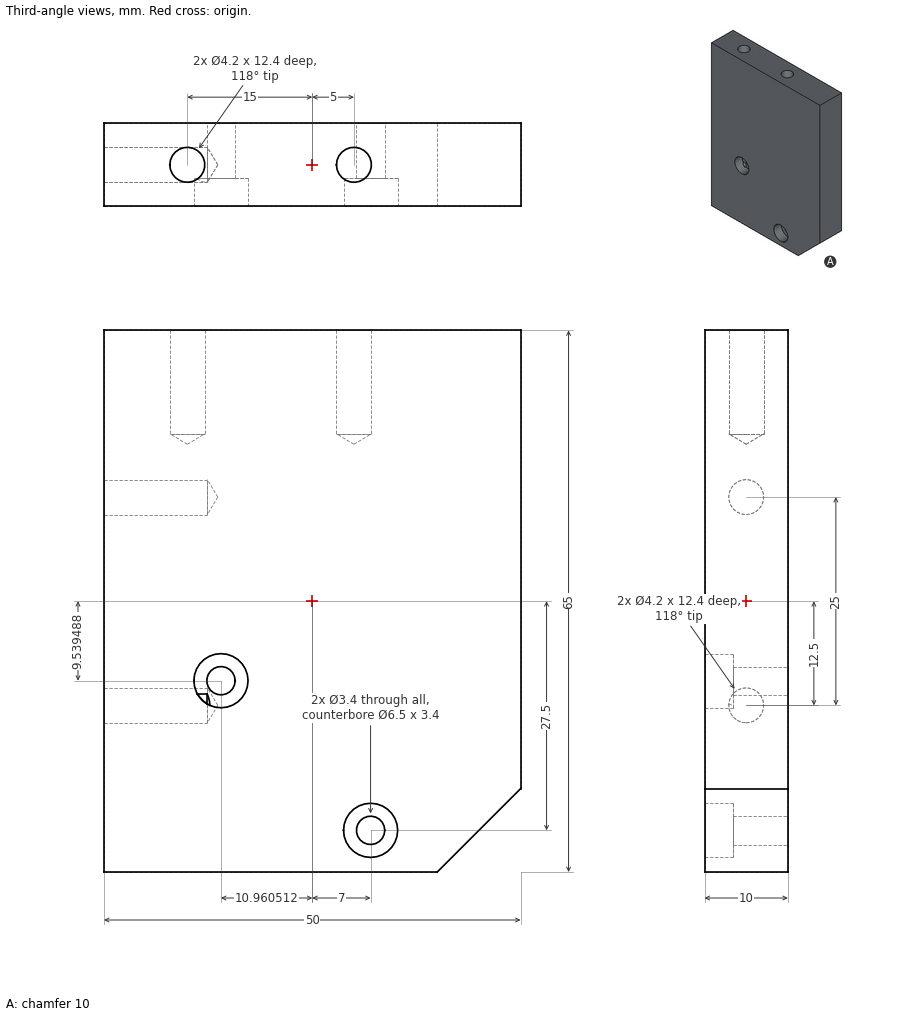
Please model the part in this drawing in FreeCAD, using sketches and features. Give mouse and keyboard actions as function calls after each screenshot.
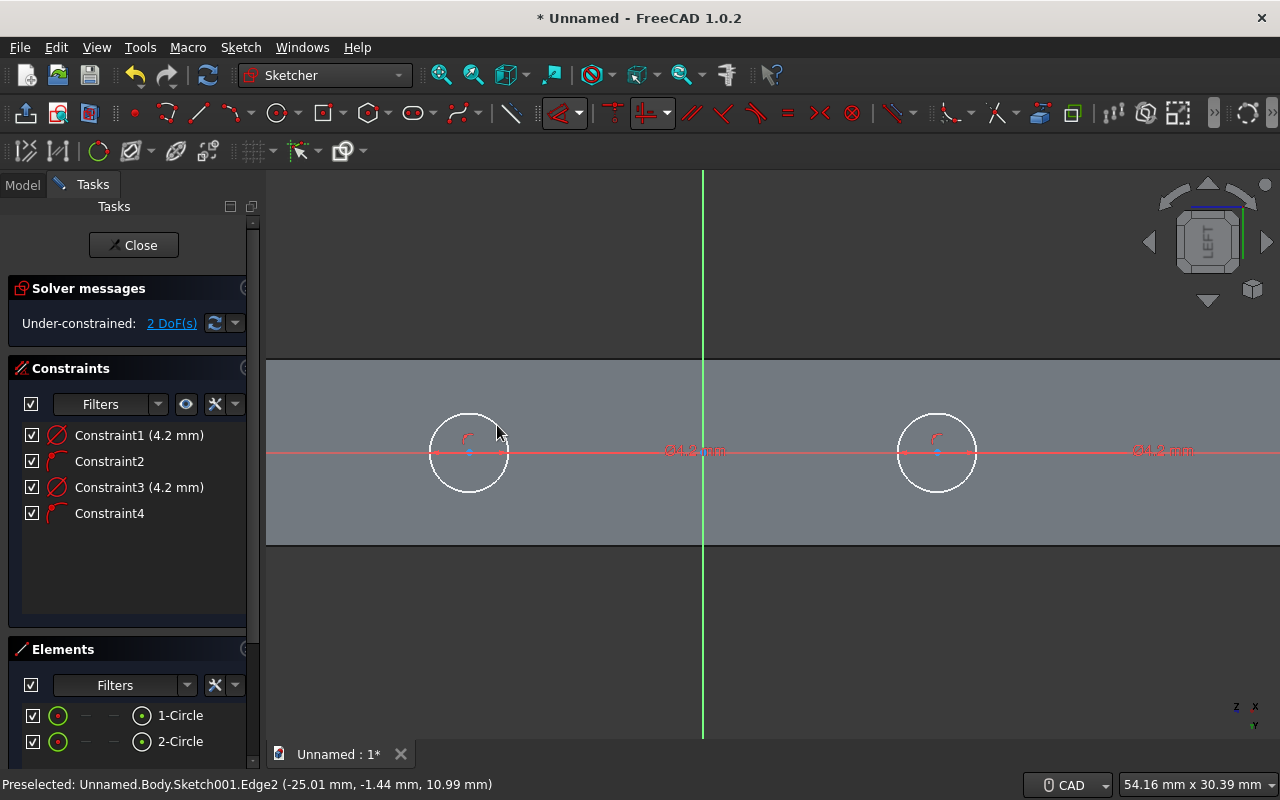
key(d)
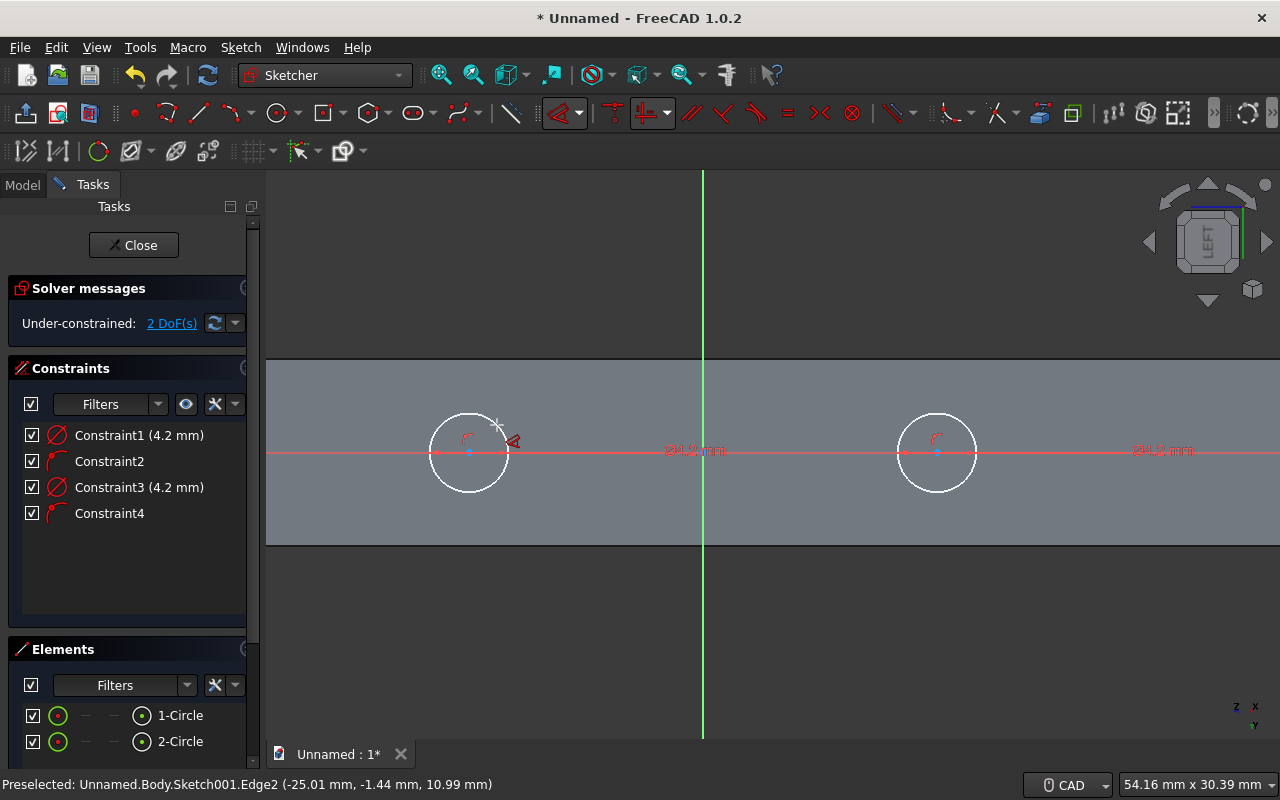
click(937, 453)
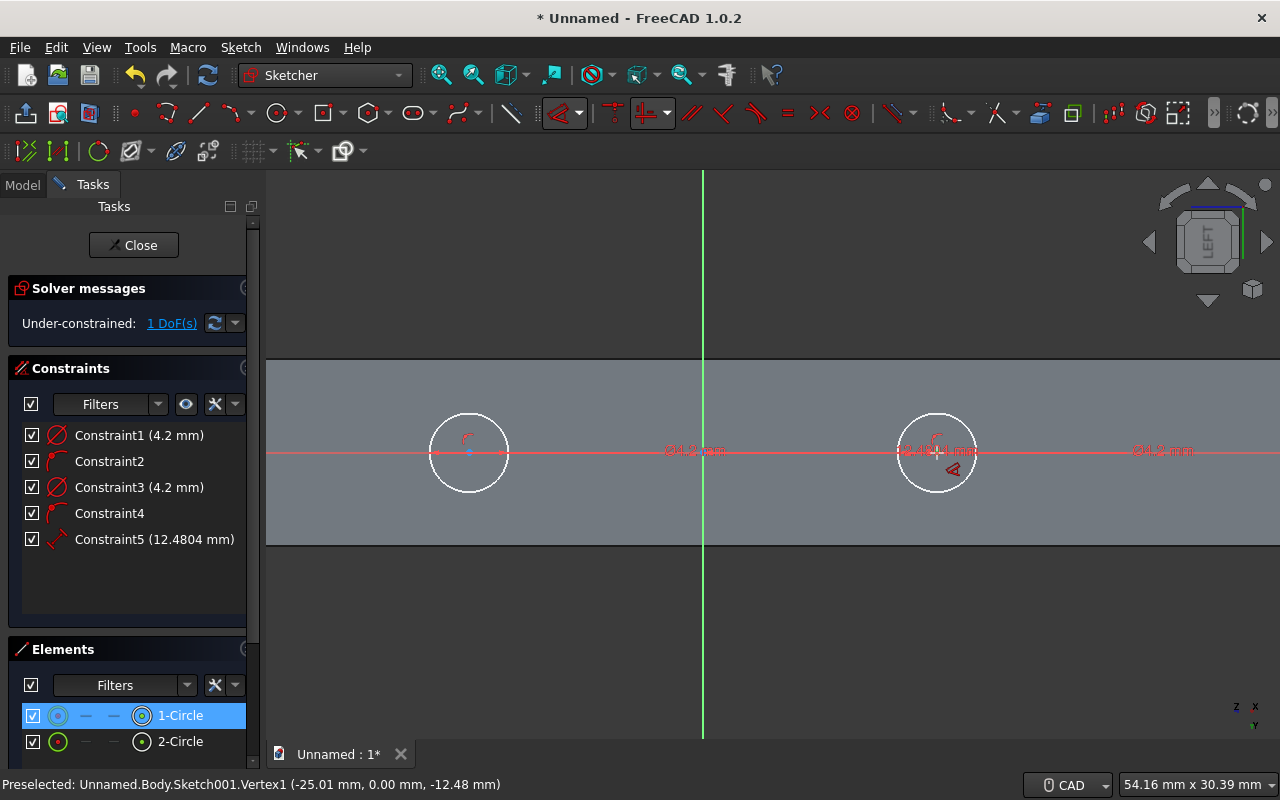
click(469, 453)
click(595, 487)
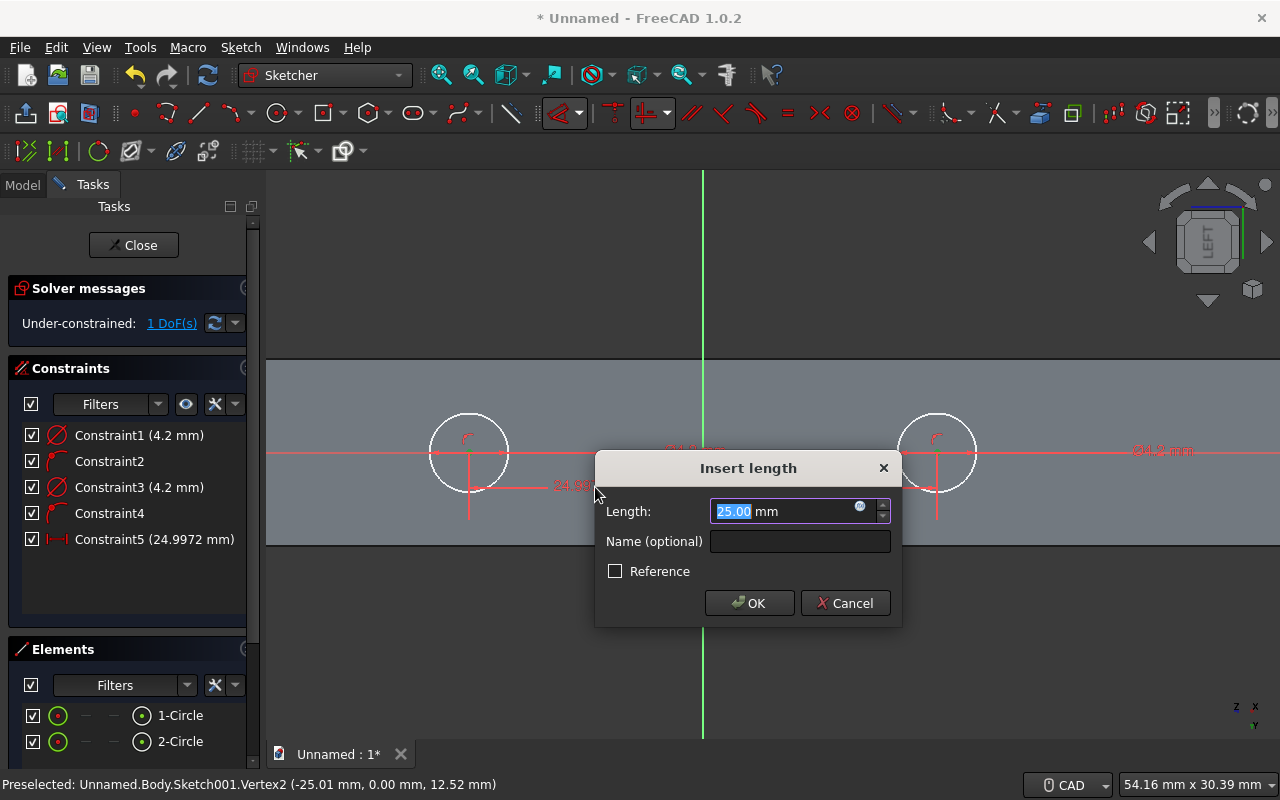
text(25)
key(Return)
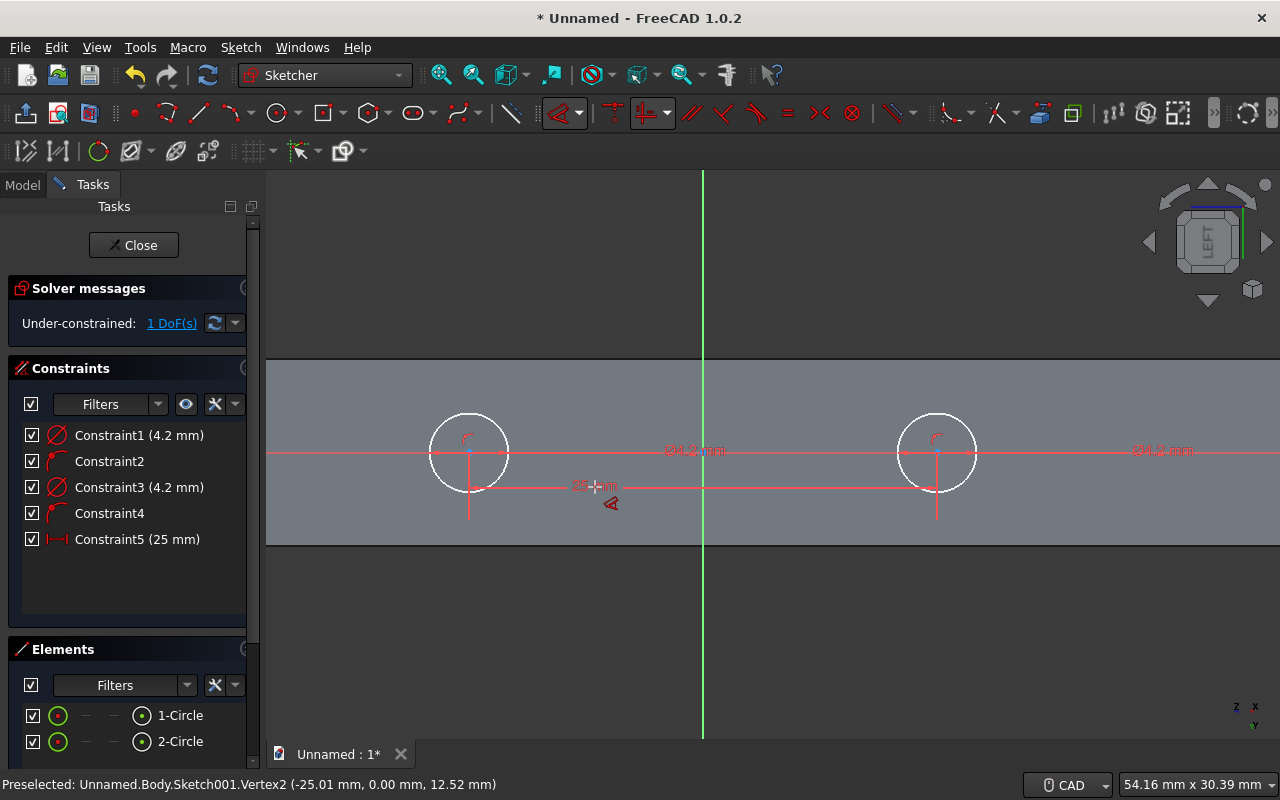
click(937, 453)
click(820, 487)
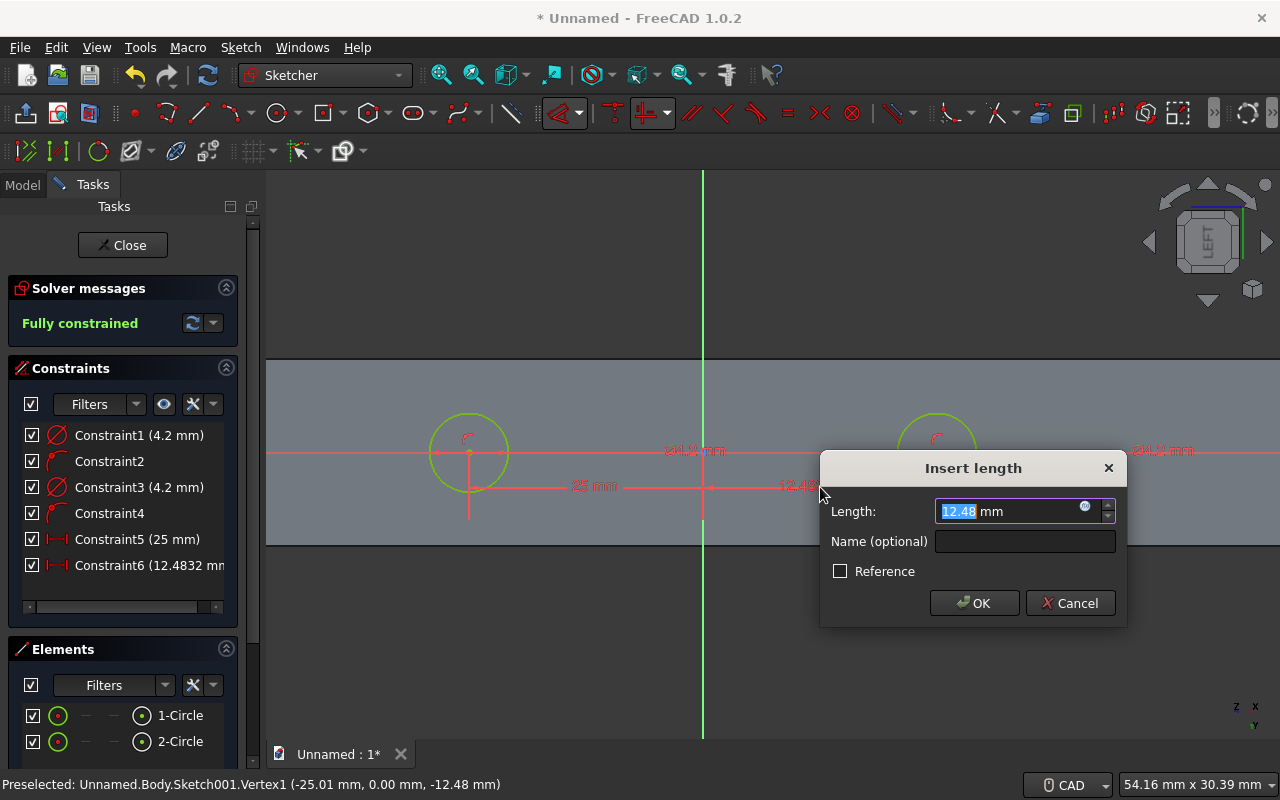
text(12.5)
key(Return)
key(Escape)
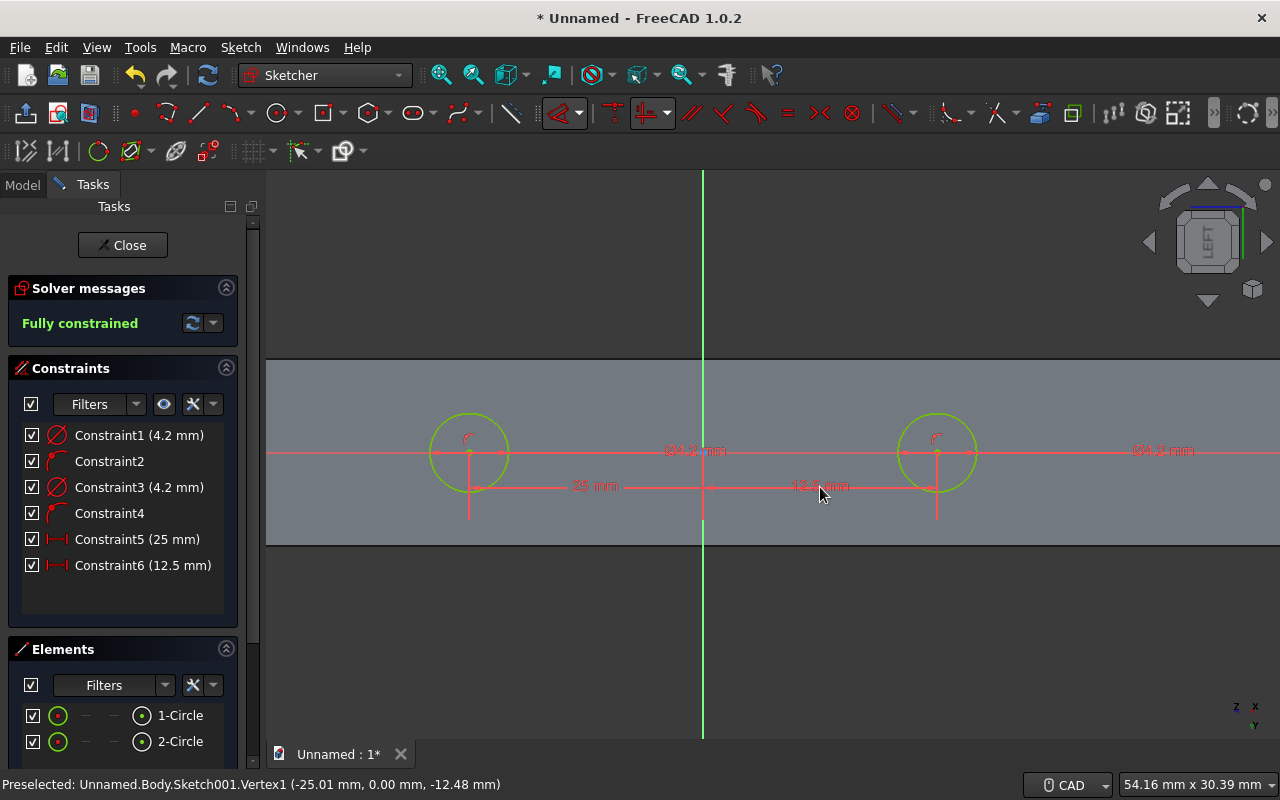
click(123, 245)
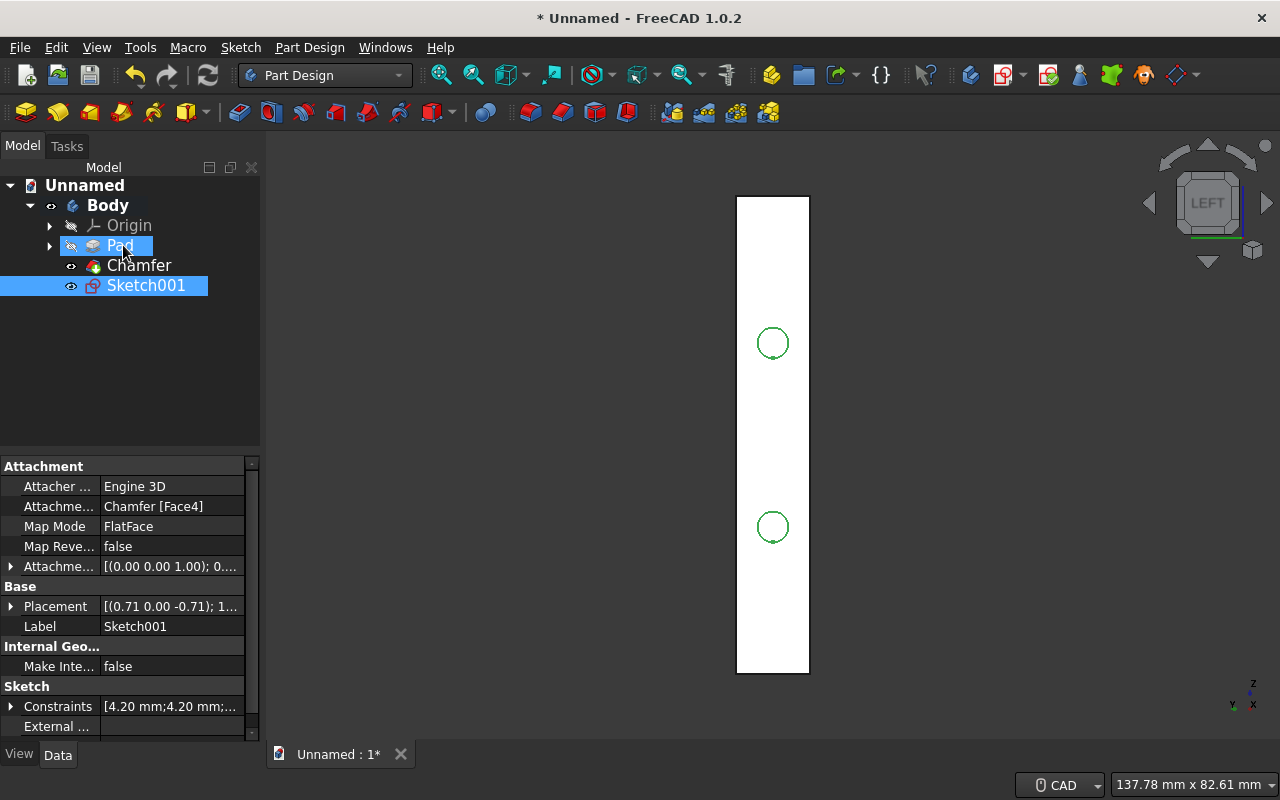
click(272, 112)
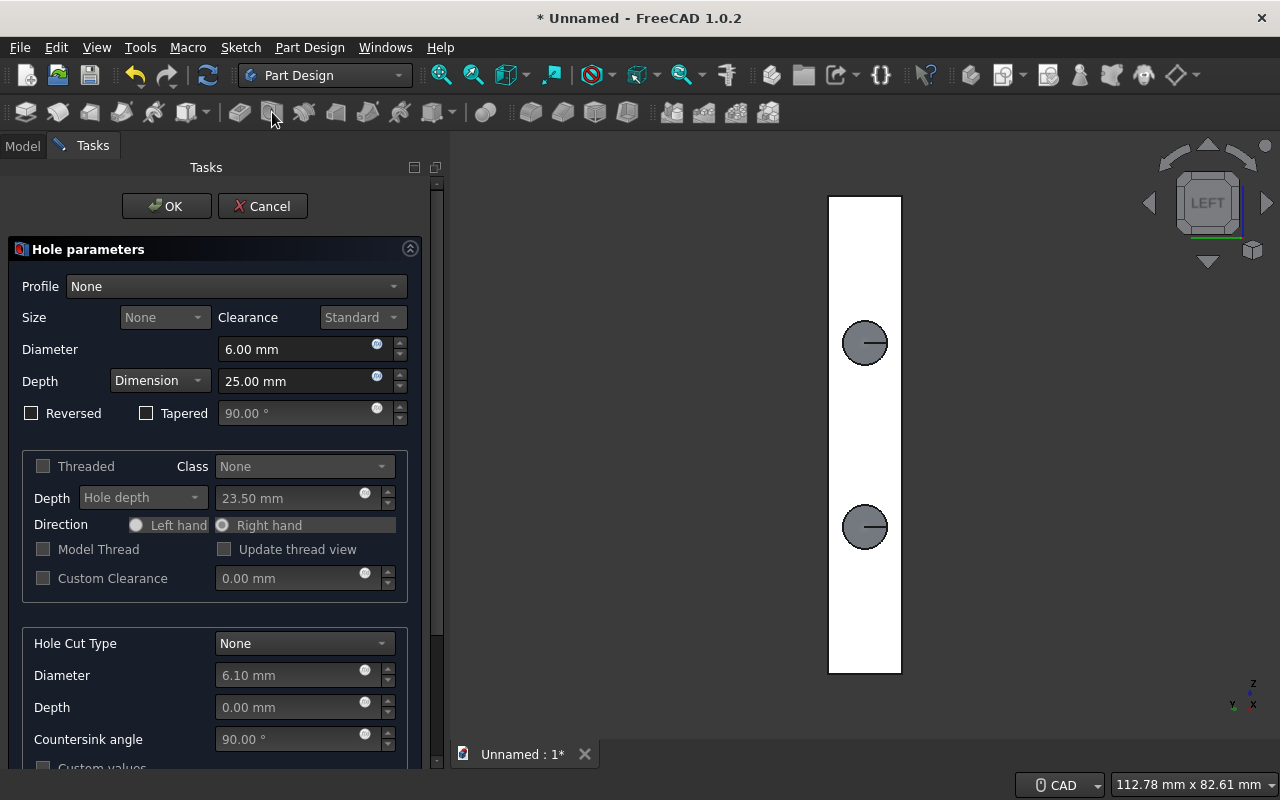
triple_click(305, 349)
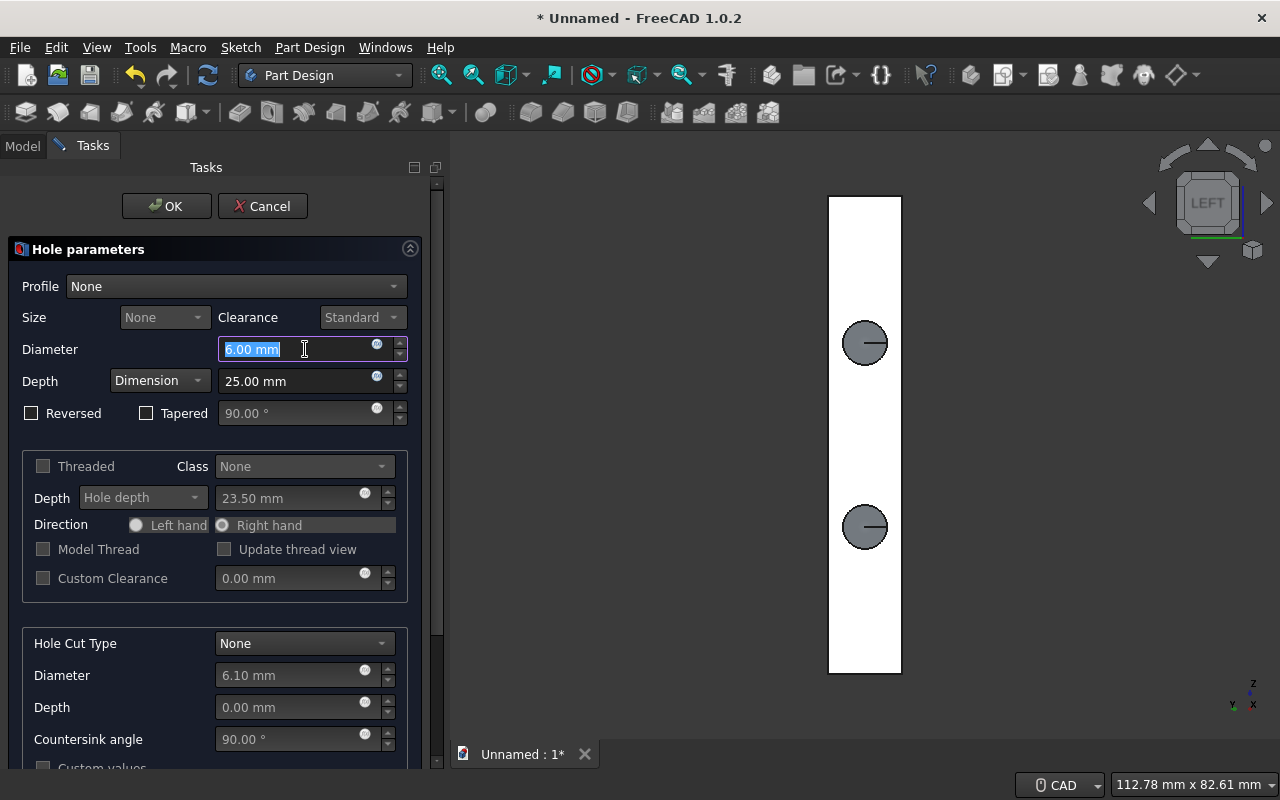
text(4.2)
key(Tab)